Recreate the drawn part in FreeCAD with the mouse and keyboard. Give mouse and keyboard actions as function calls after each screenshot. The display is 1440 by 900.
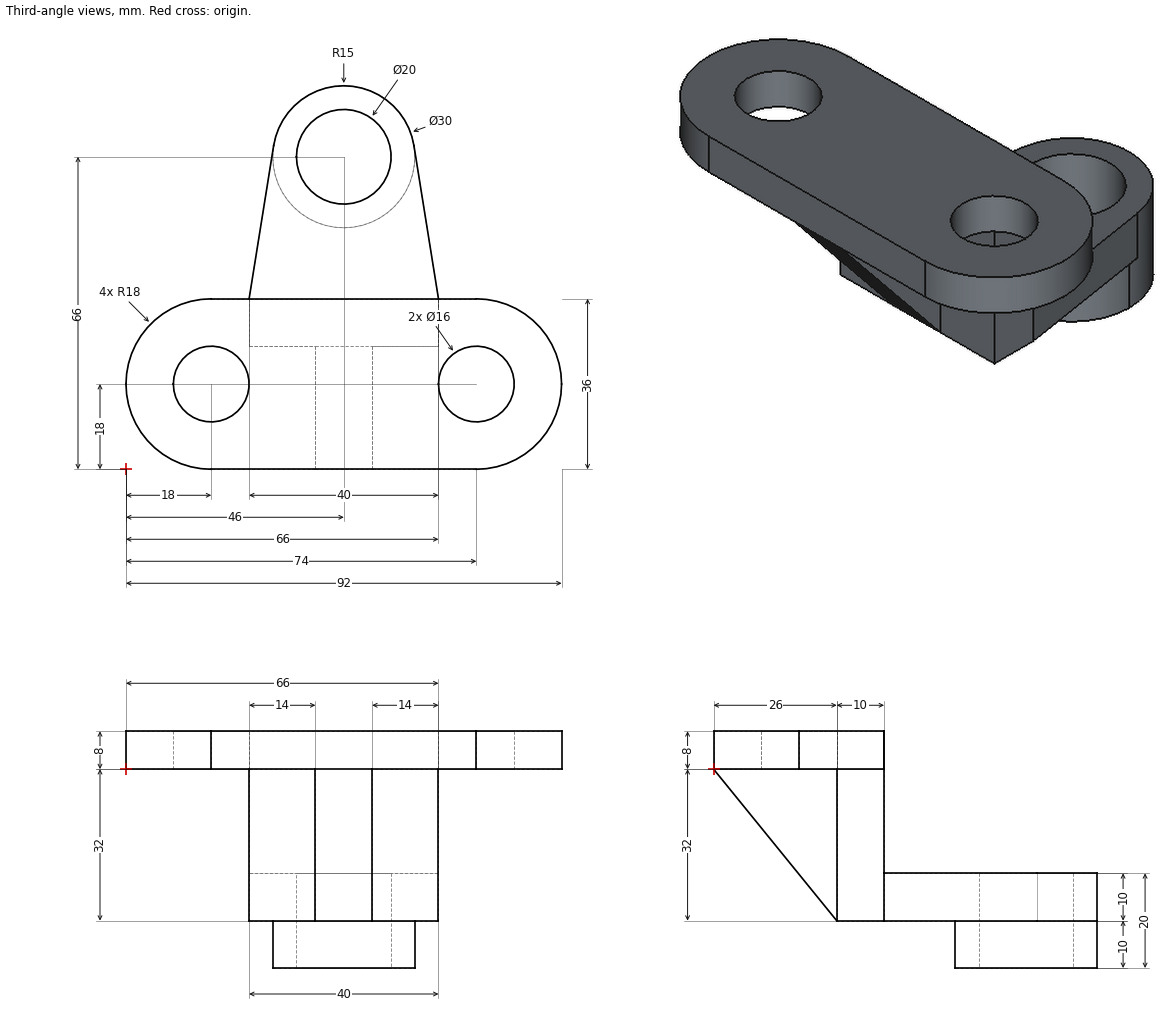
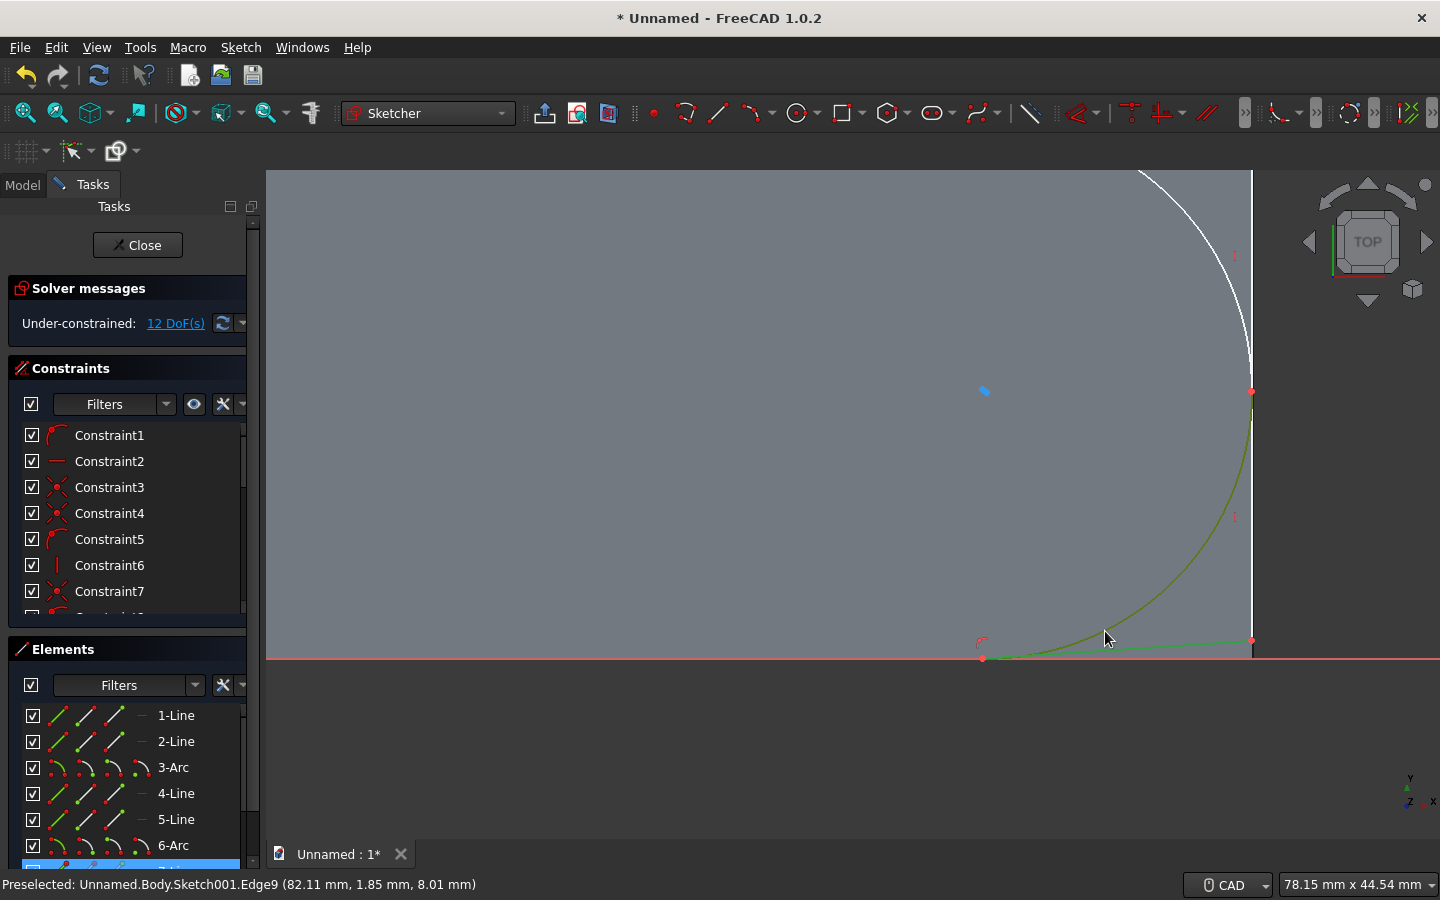
key(t)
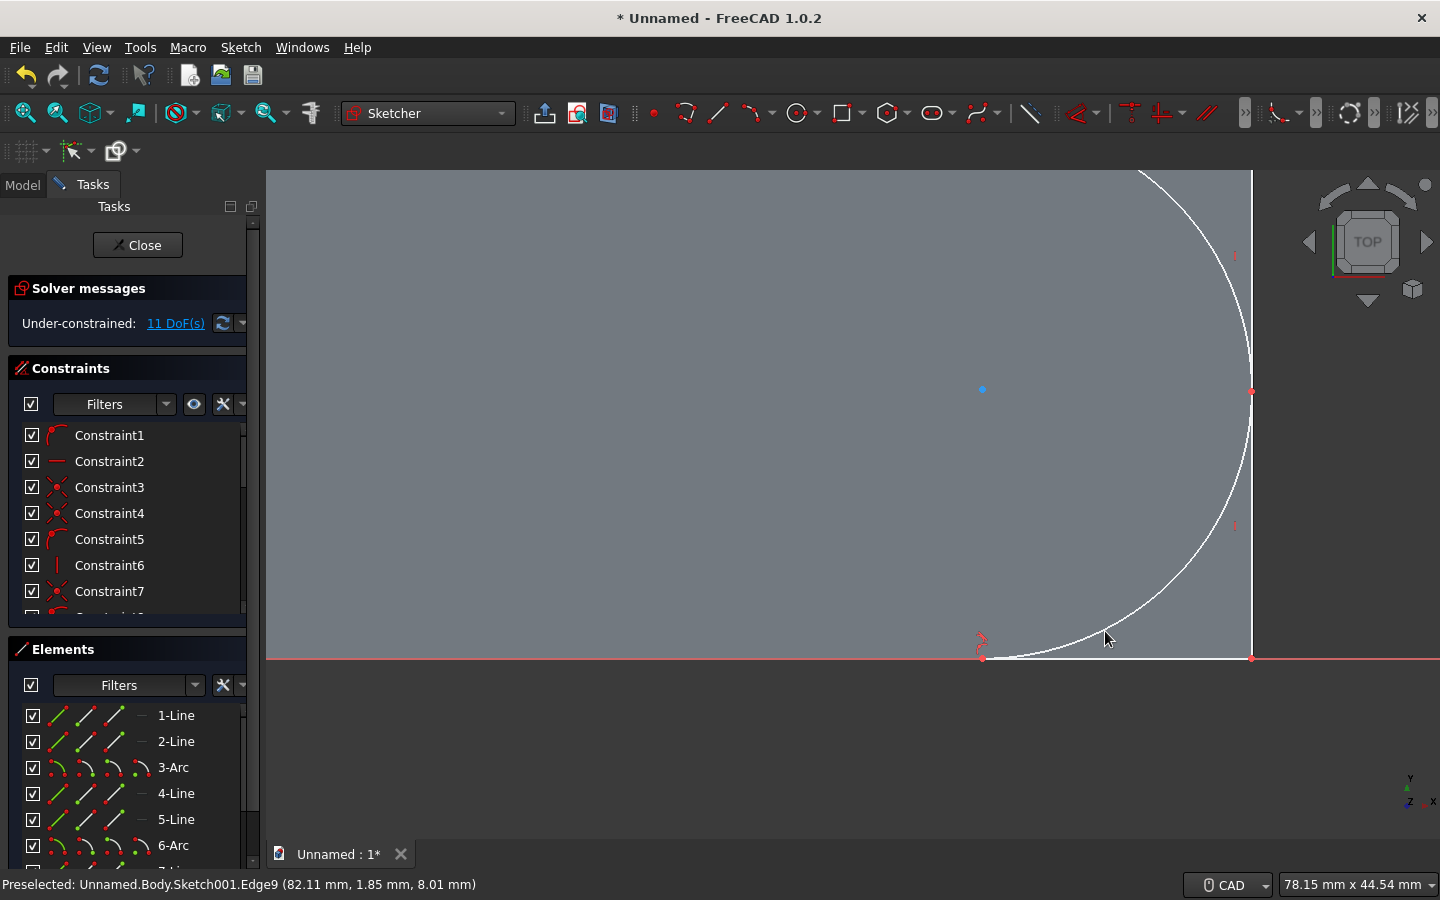
click(1252, 579)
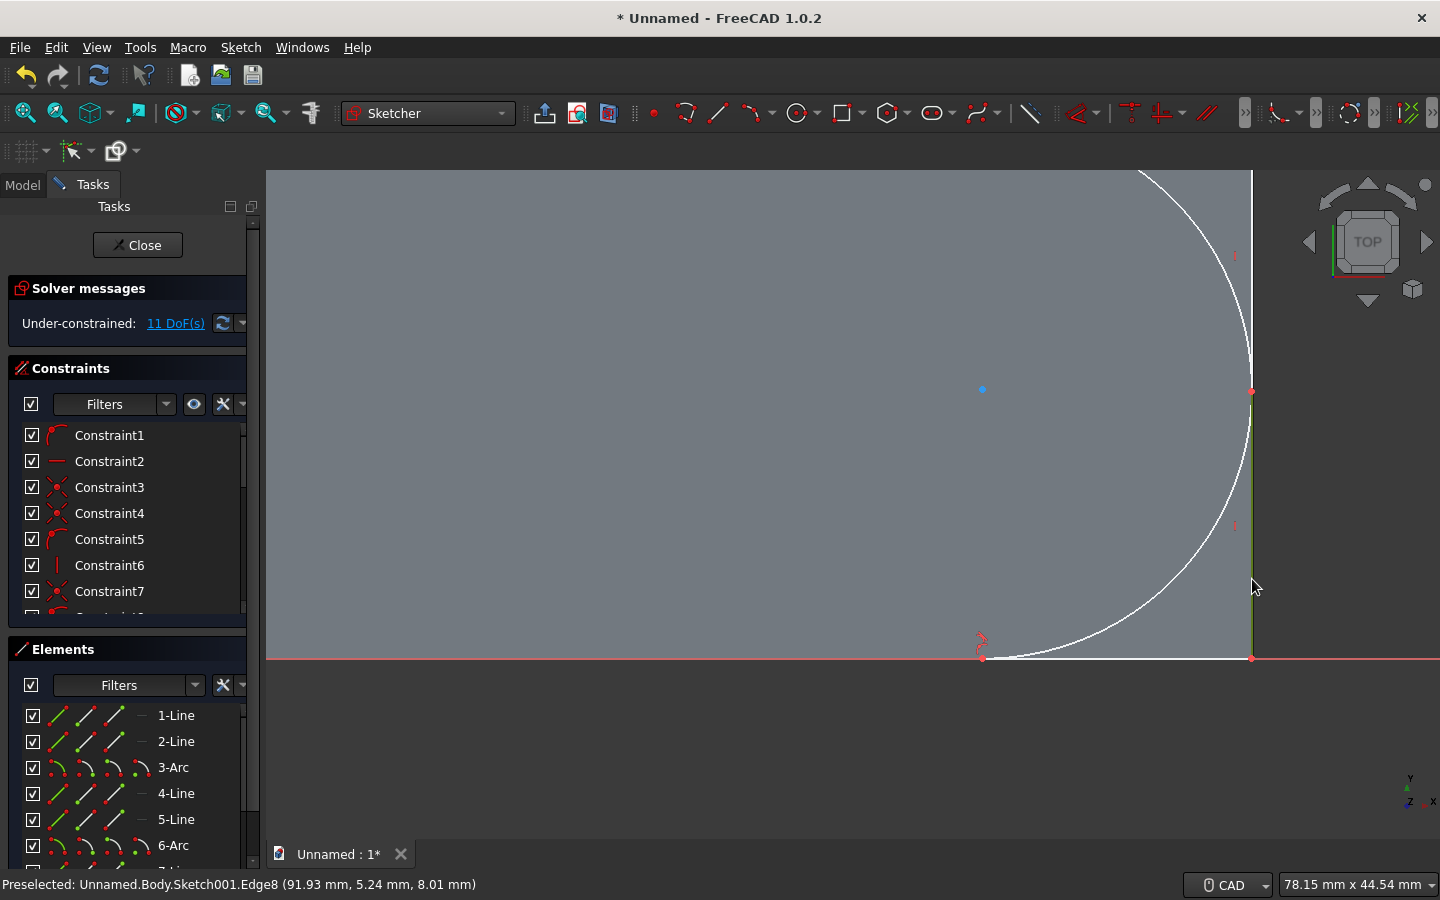
click(1104, 630)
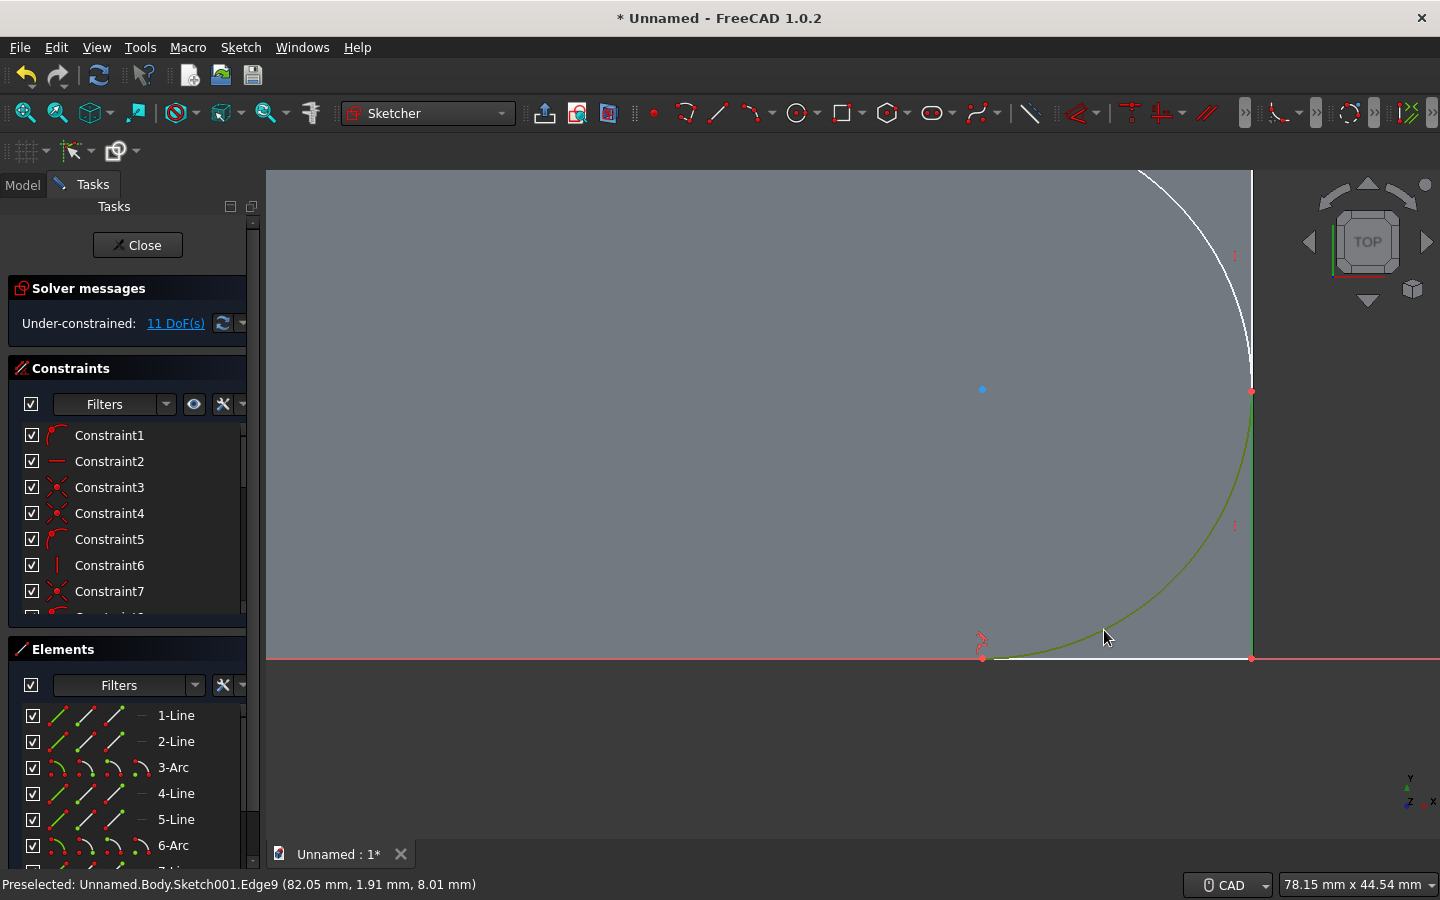
key(t)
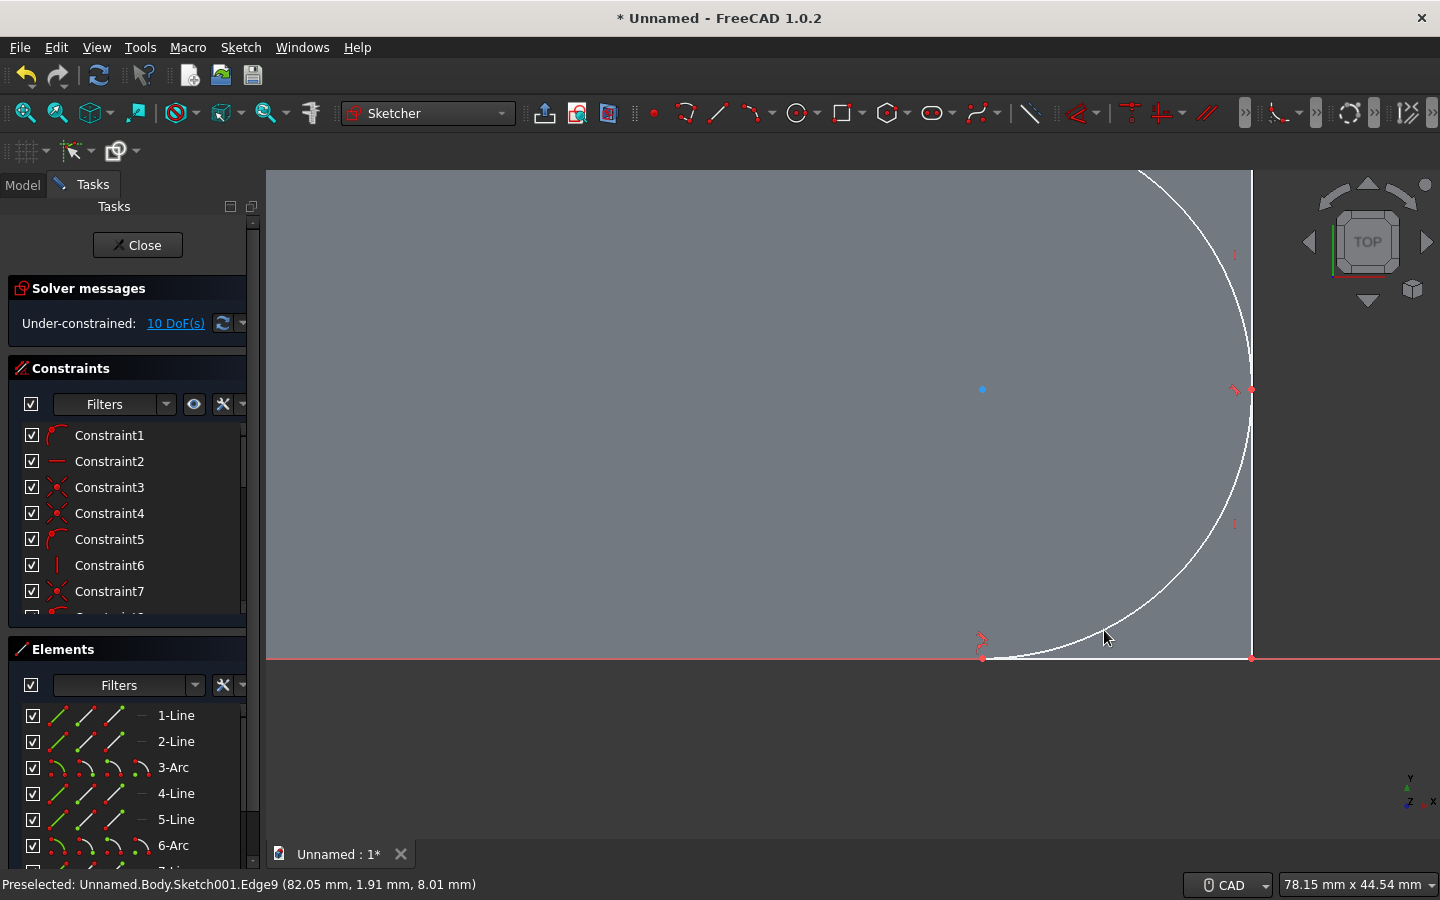
click(1252, 578)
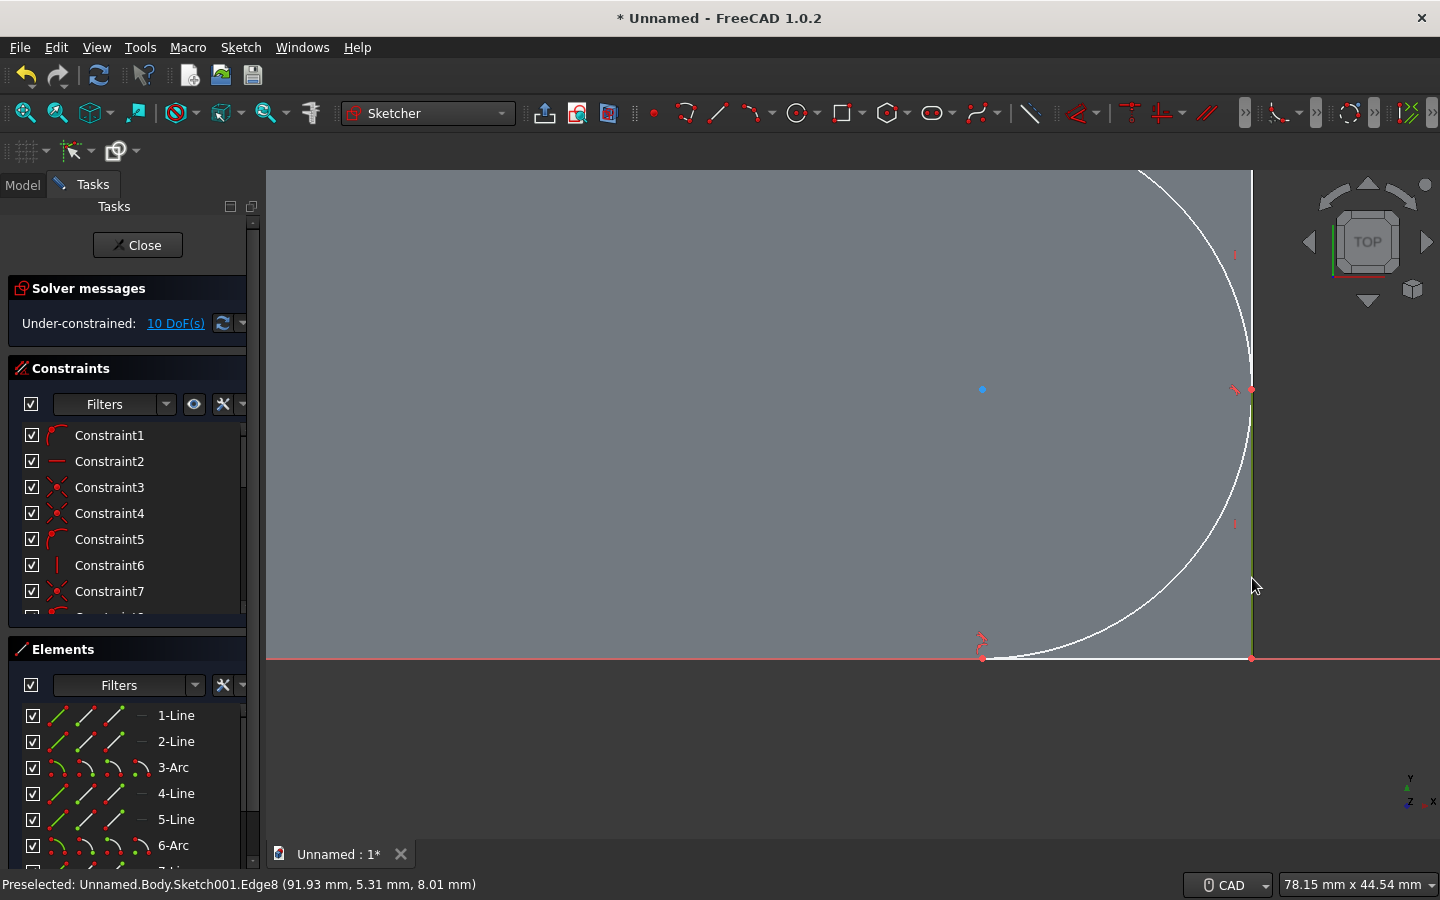
click(1222, 267)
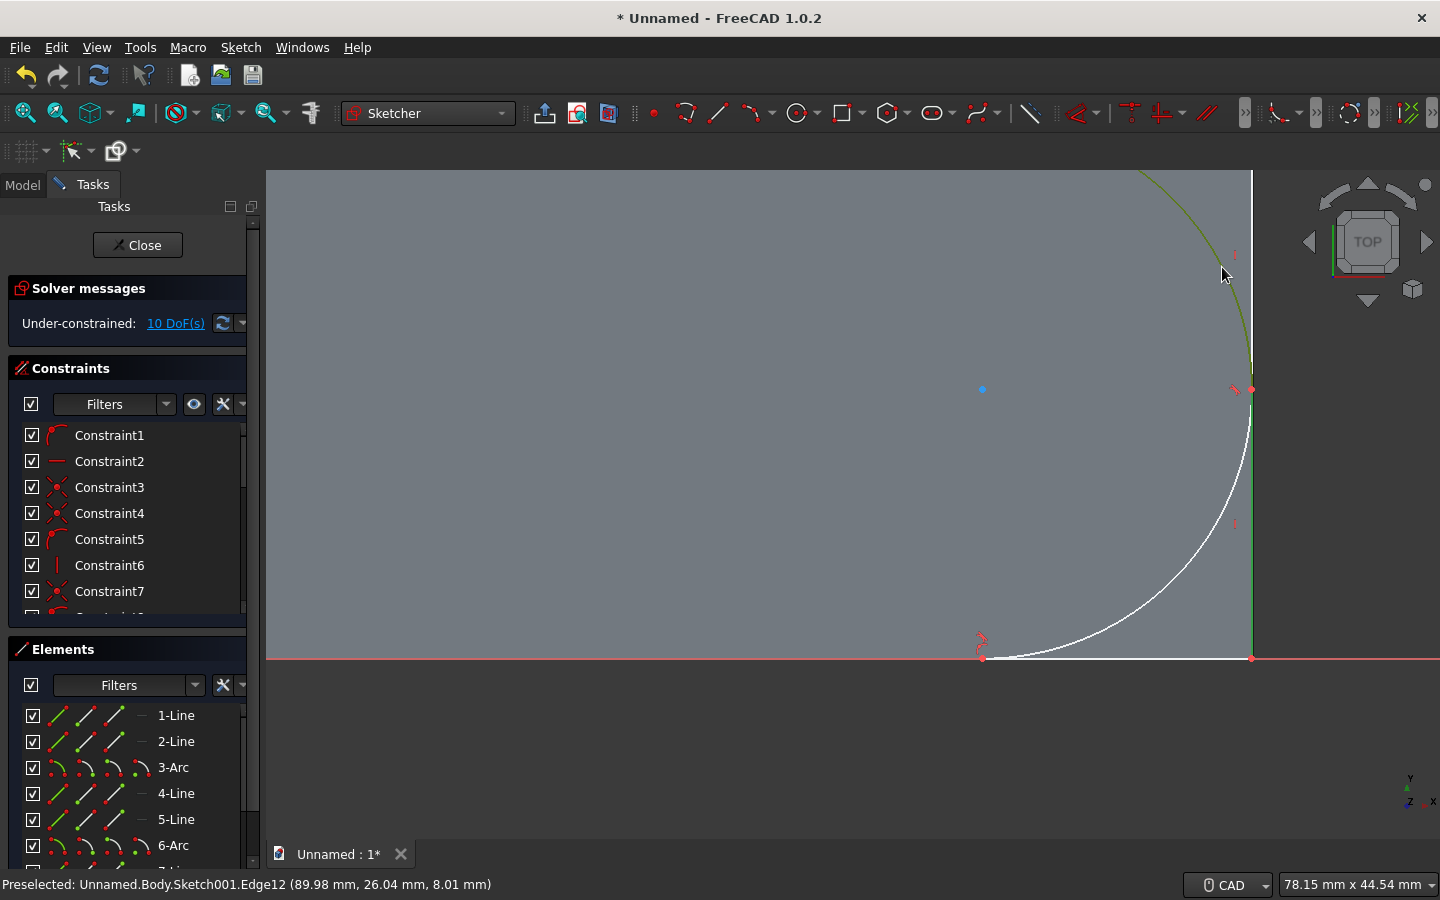
key(t)